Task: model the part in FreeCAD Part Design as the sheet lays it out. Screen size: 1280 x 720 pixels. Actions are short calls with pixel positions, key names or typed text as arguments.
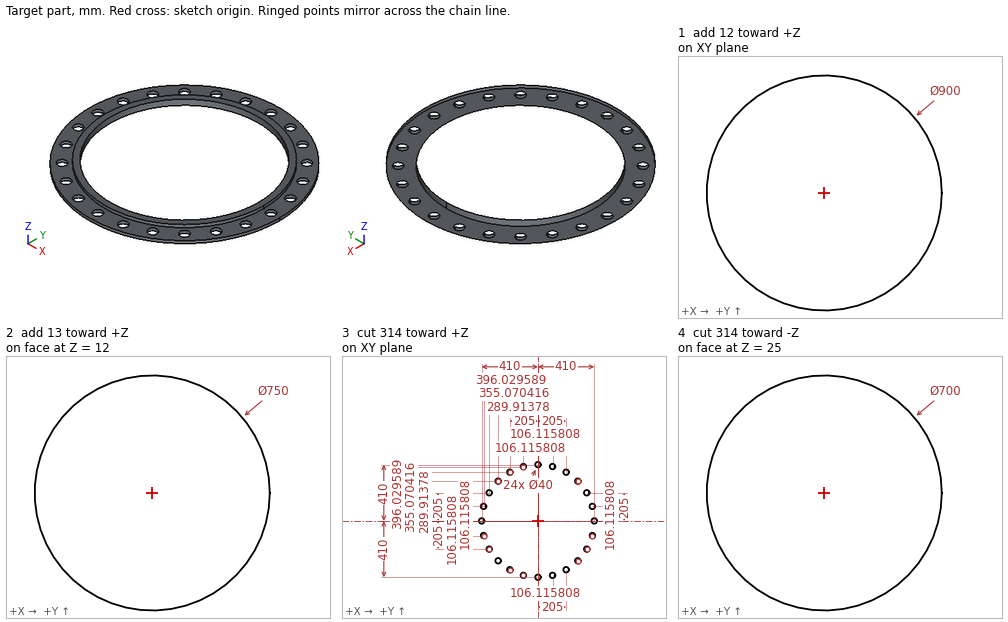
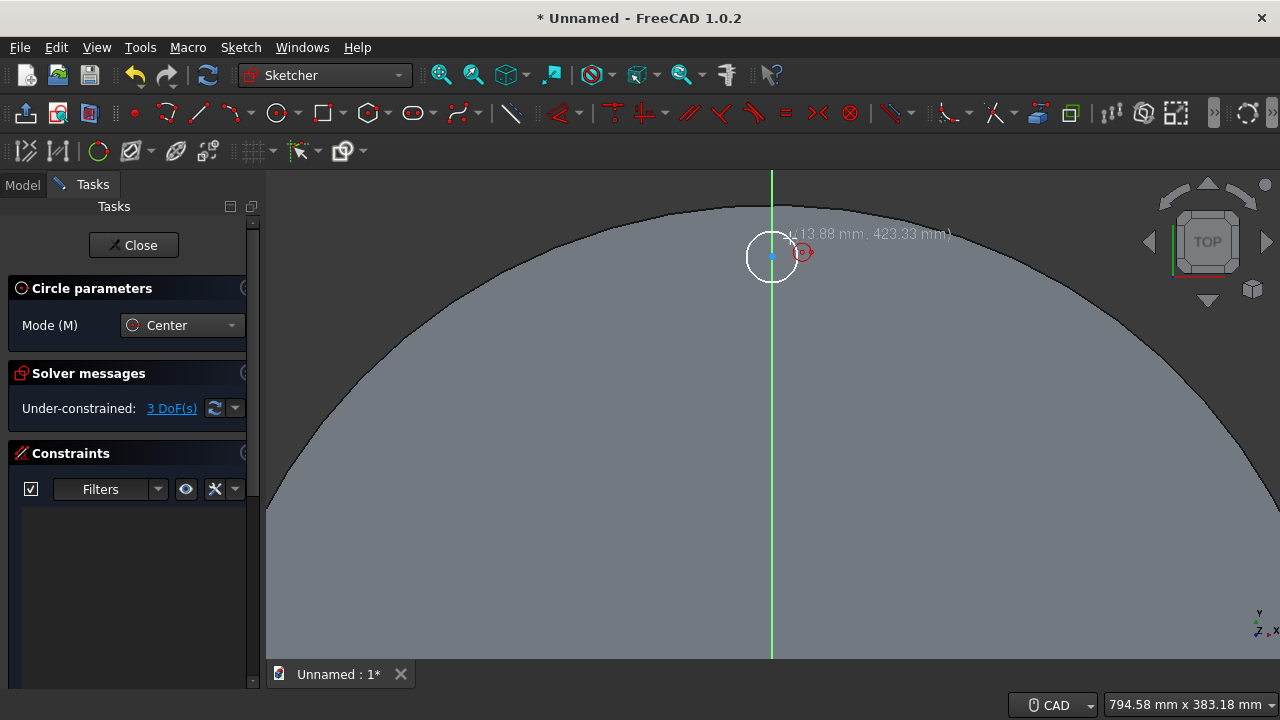
click(637, 274)
click(655, 256)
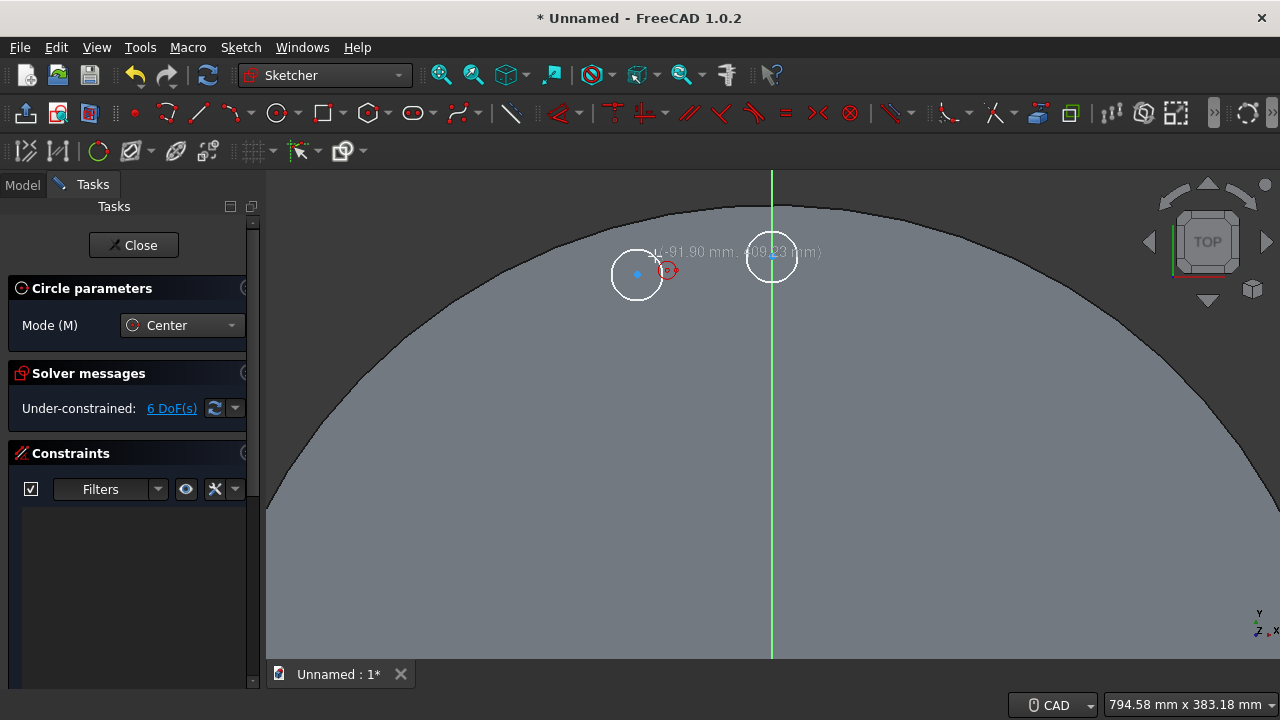
click(511, 326)
click(529, 308)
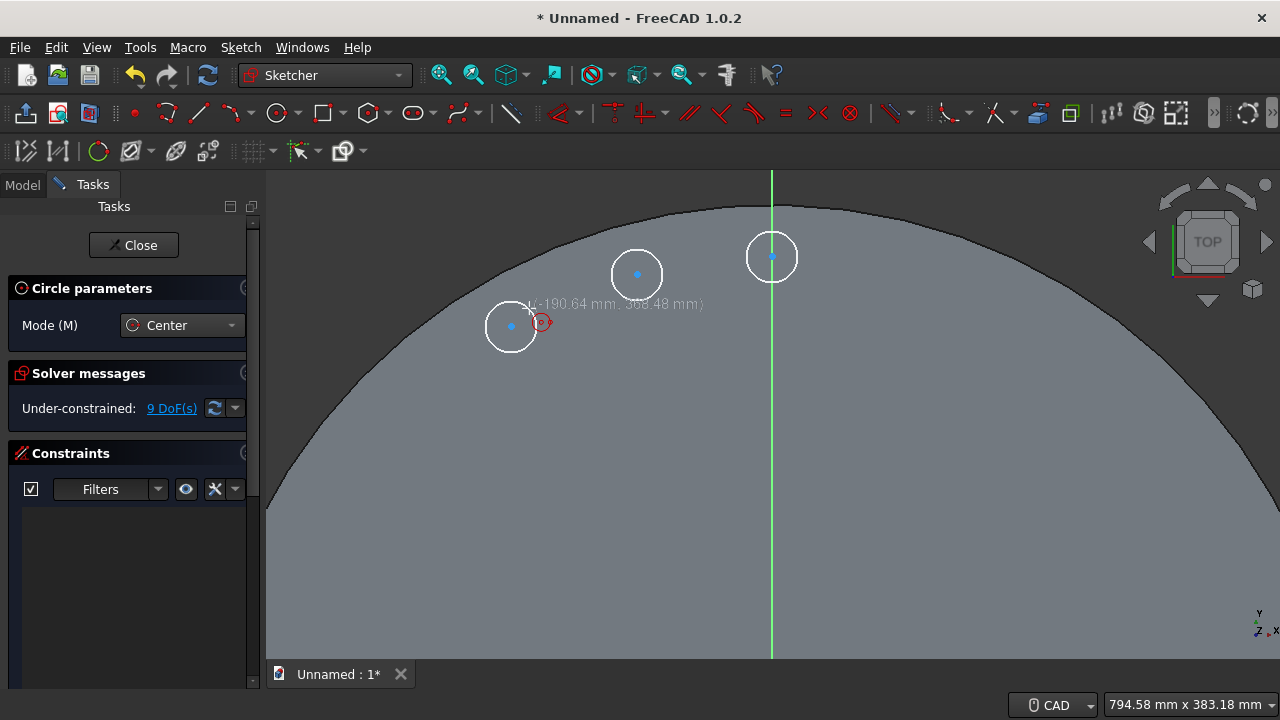
click(402, 409)
click(420, 391)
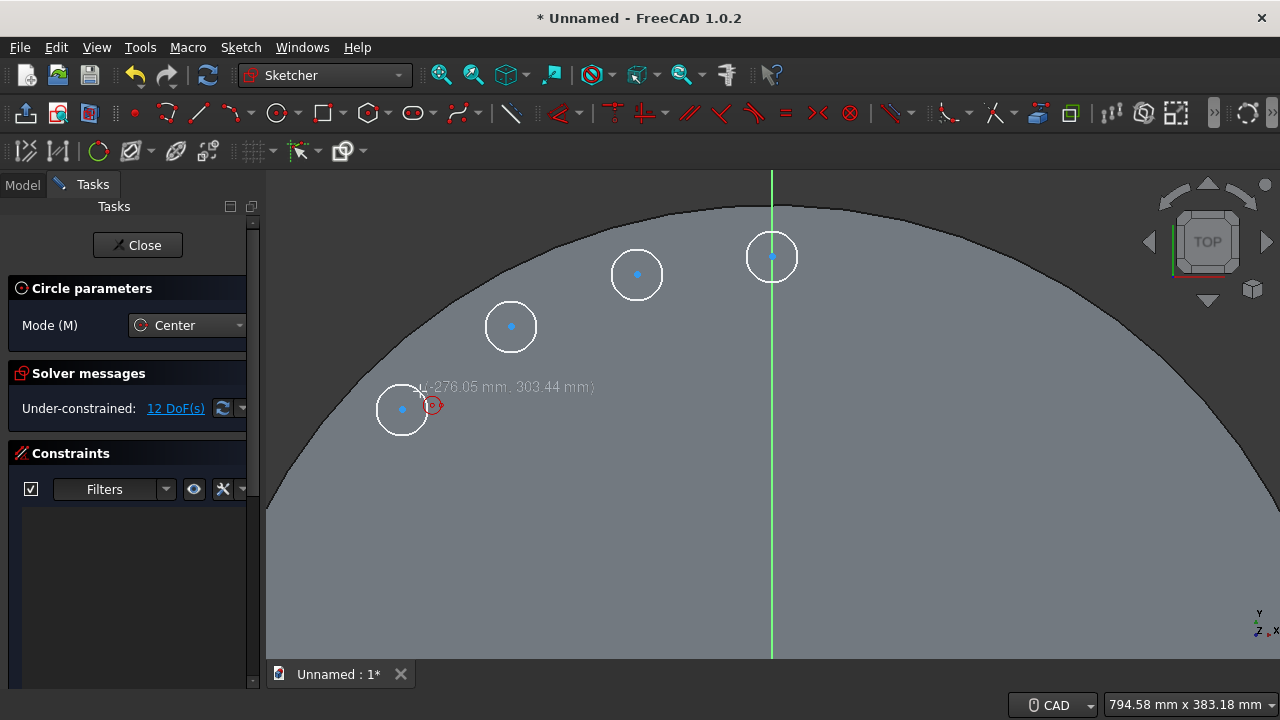
click(319, 518)
click(337, 500)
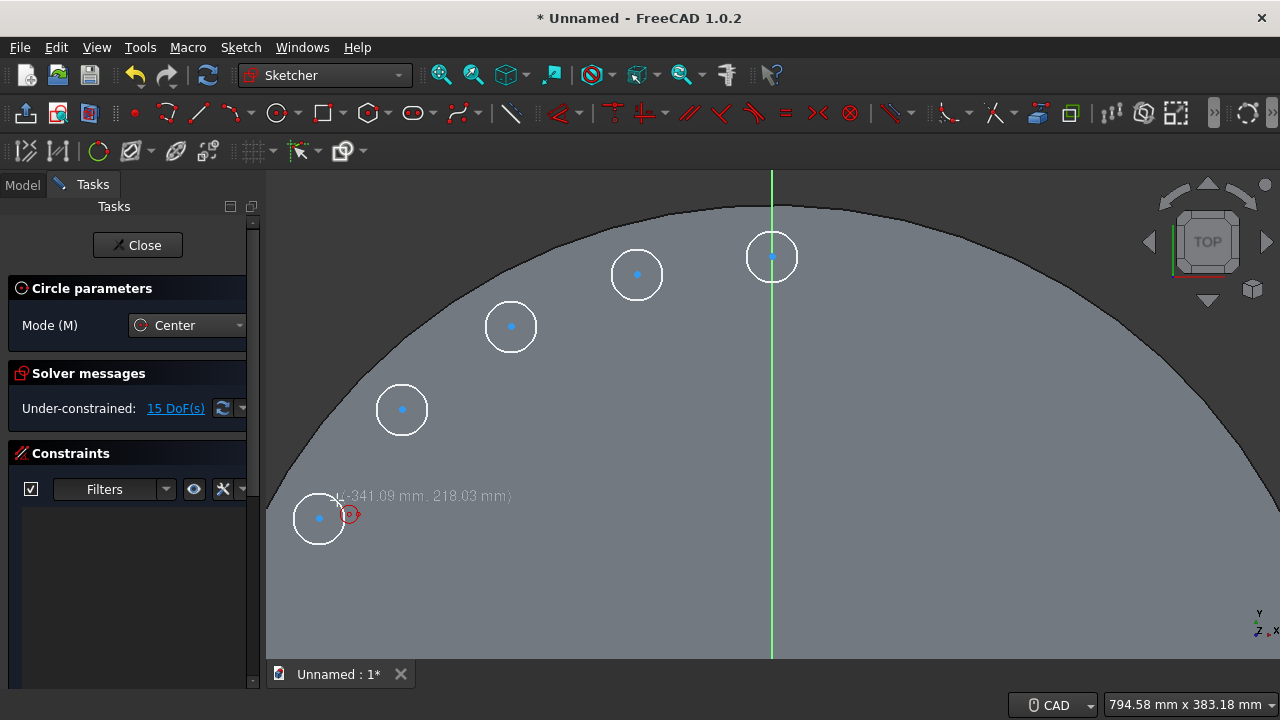
scroll(675, 257, down, 6)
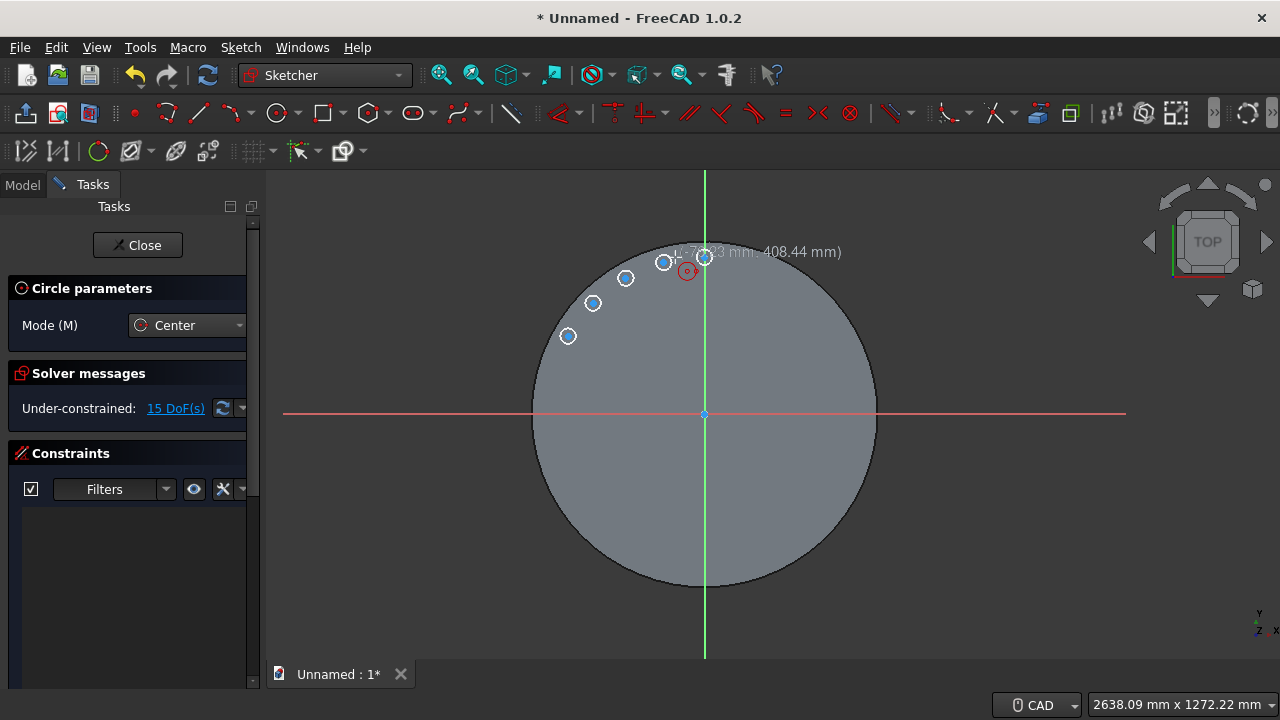
scroll(552, 374, up, 6)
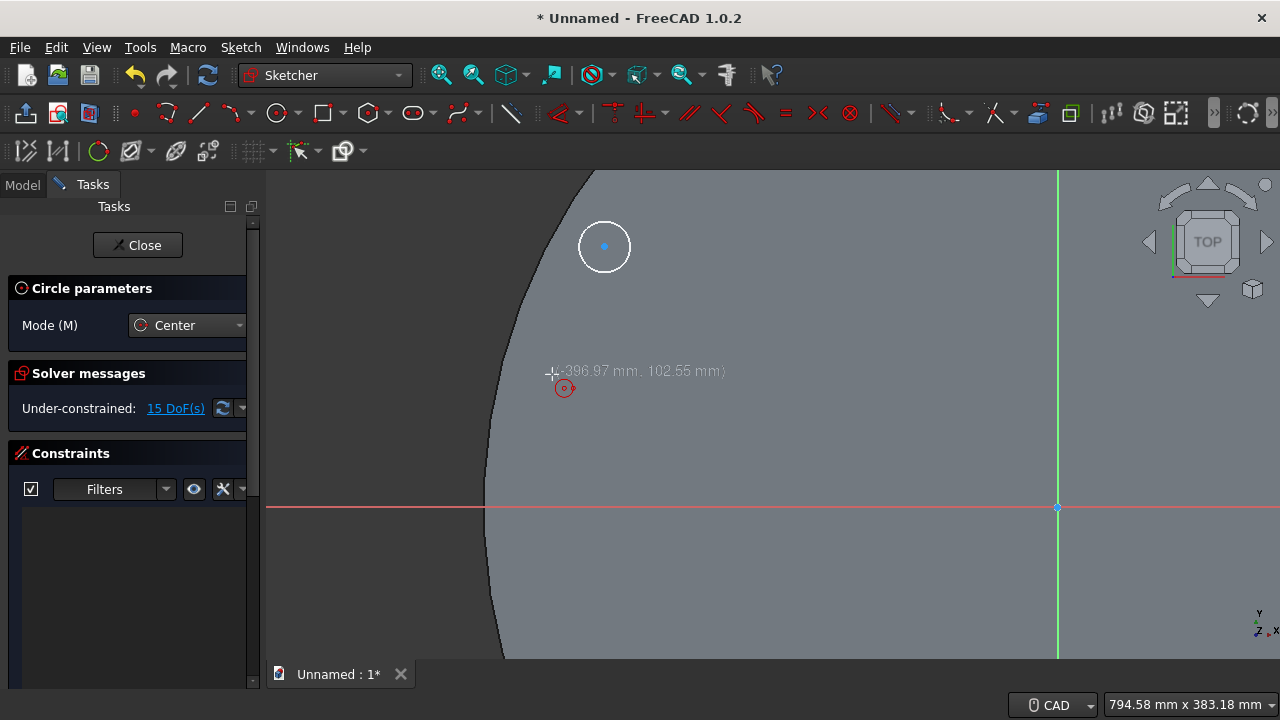
click(553, 372)
click(571, 354)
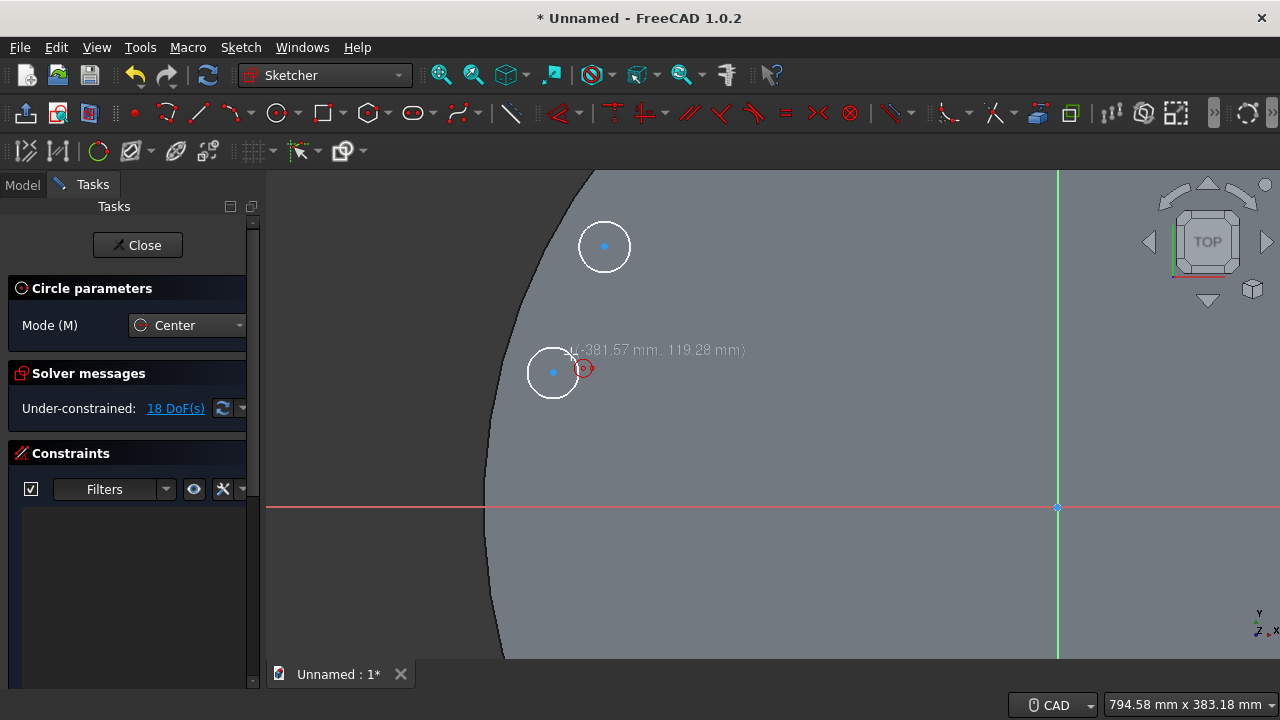
click(535, 507)
click(553, 489)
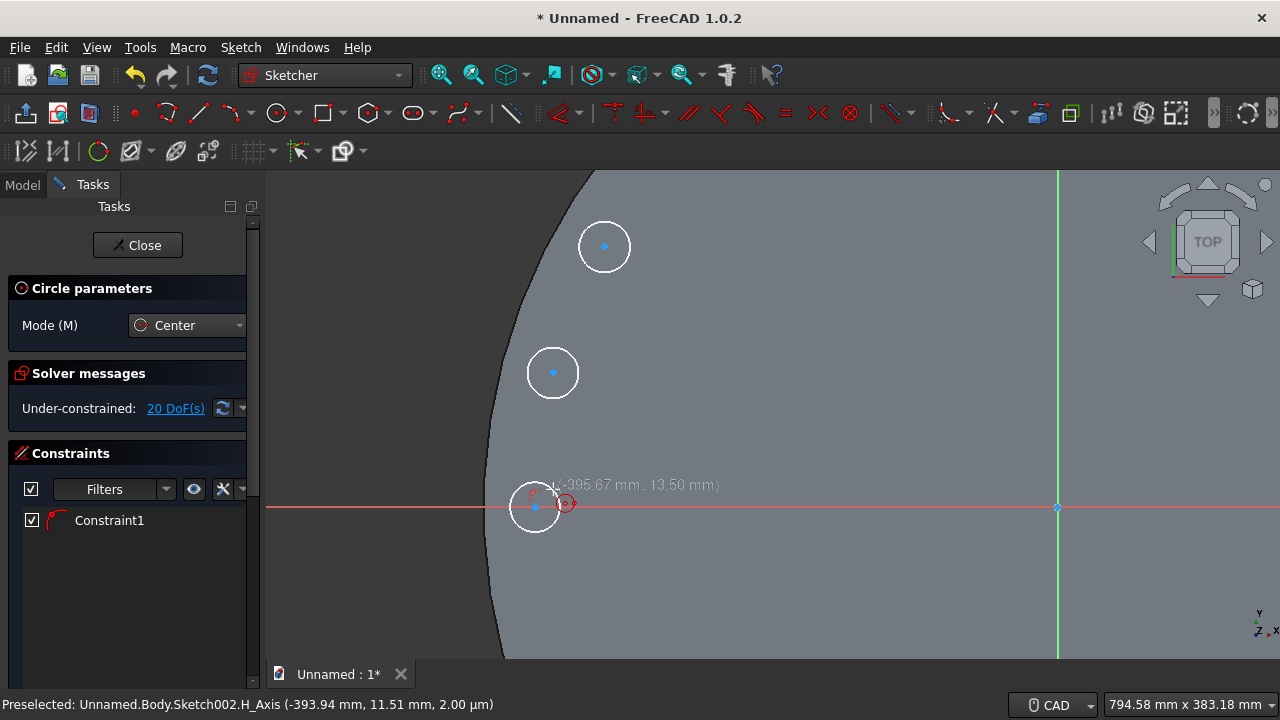
scroll(552, 375, down, 6)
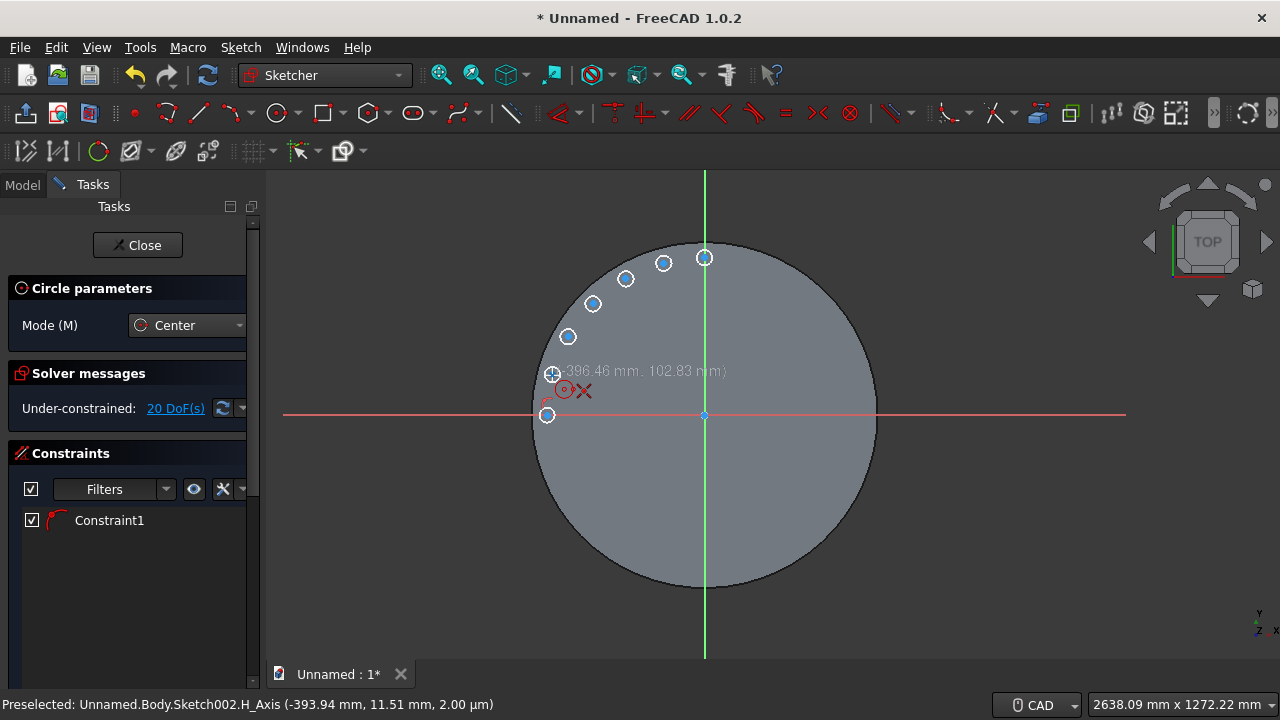
scroll(552, 456, up, 6)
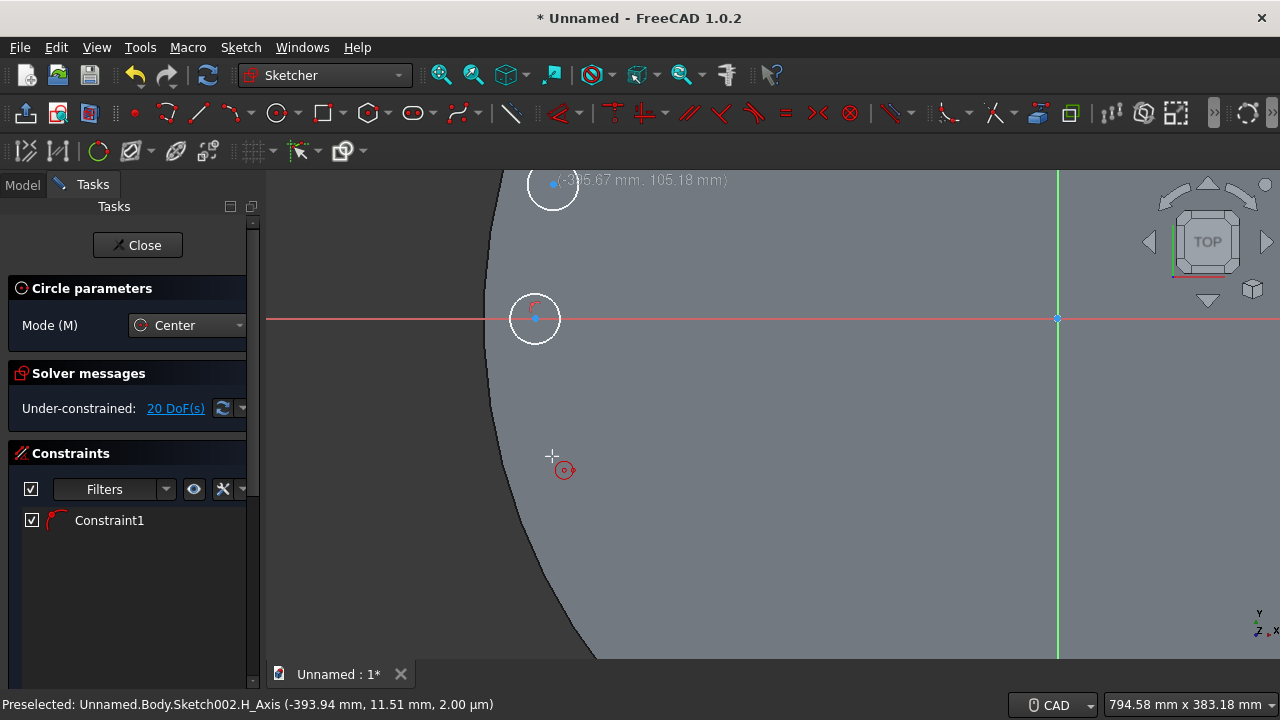
click(553, 454)
click(571, 436)